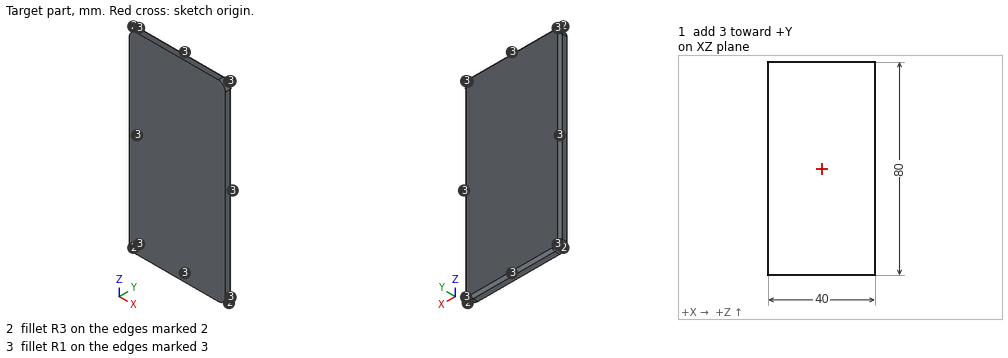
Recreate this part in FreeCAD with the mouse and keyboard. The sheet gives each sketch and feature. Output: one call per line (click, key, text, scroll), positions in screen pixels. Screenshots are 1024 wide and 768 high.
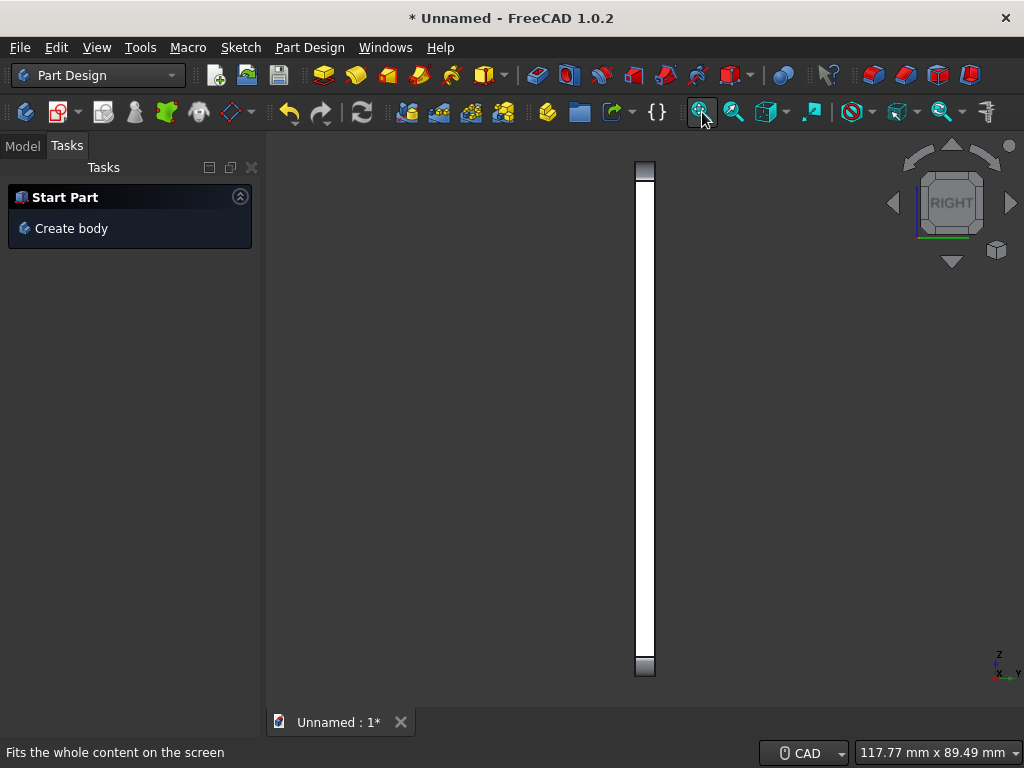
key(5)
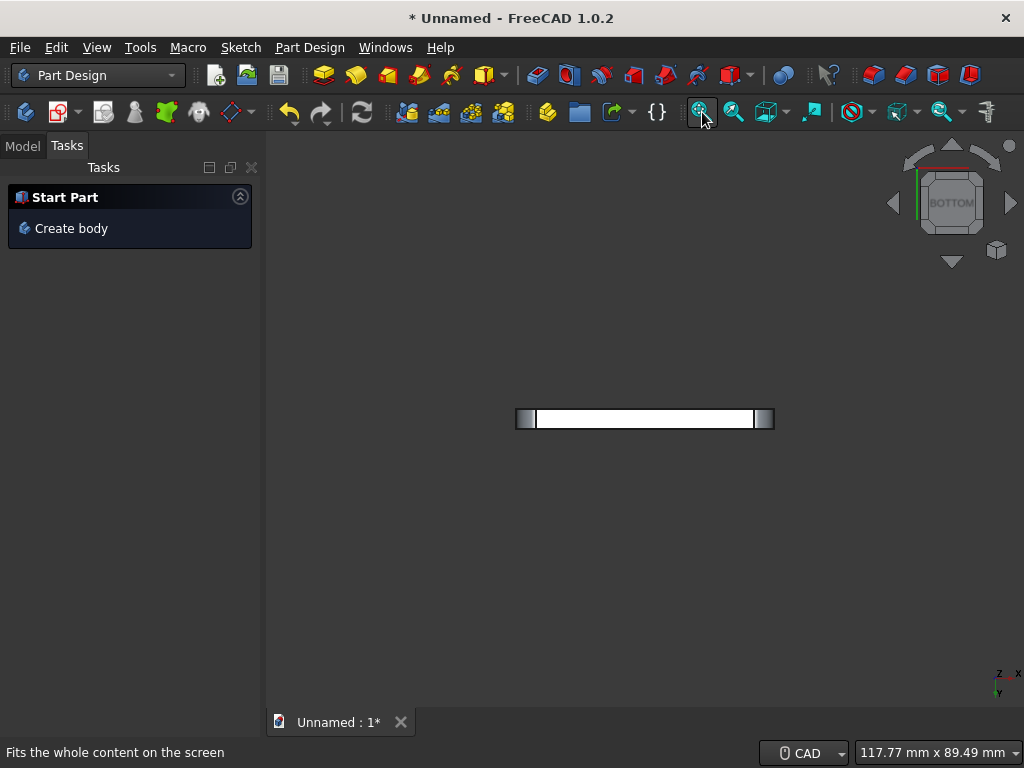
click(702, 112)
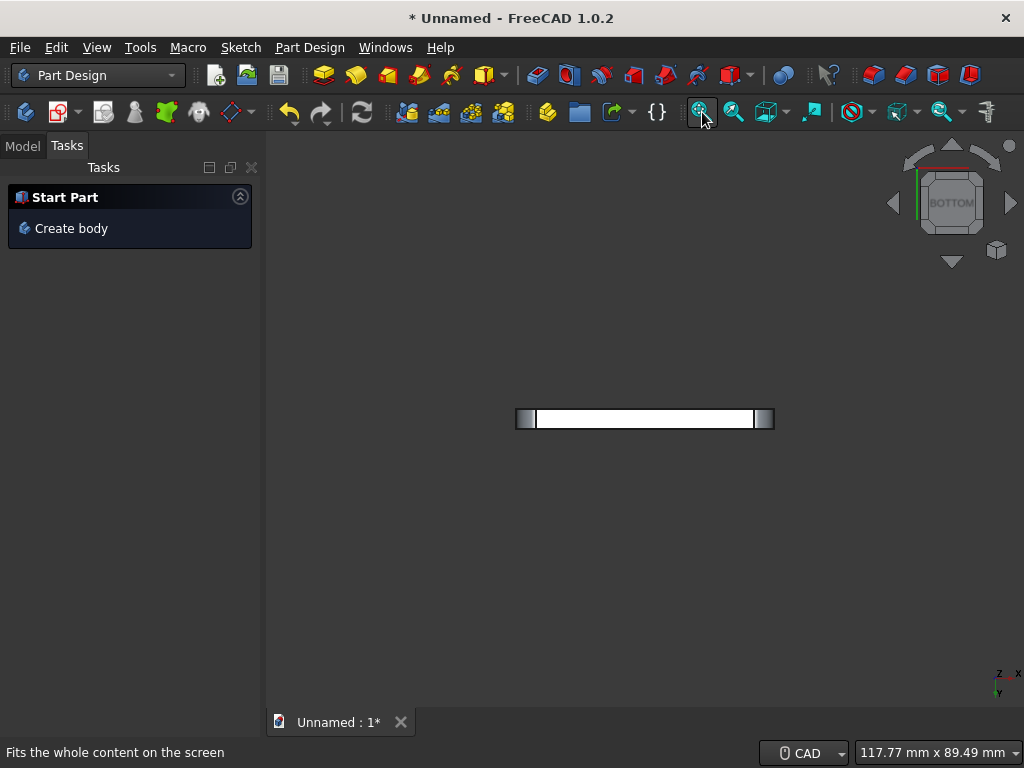
key(4)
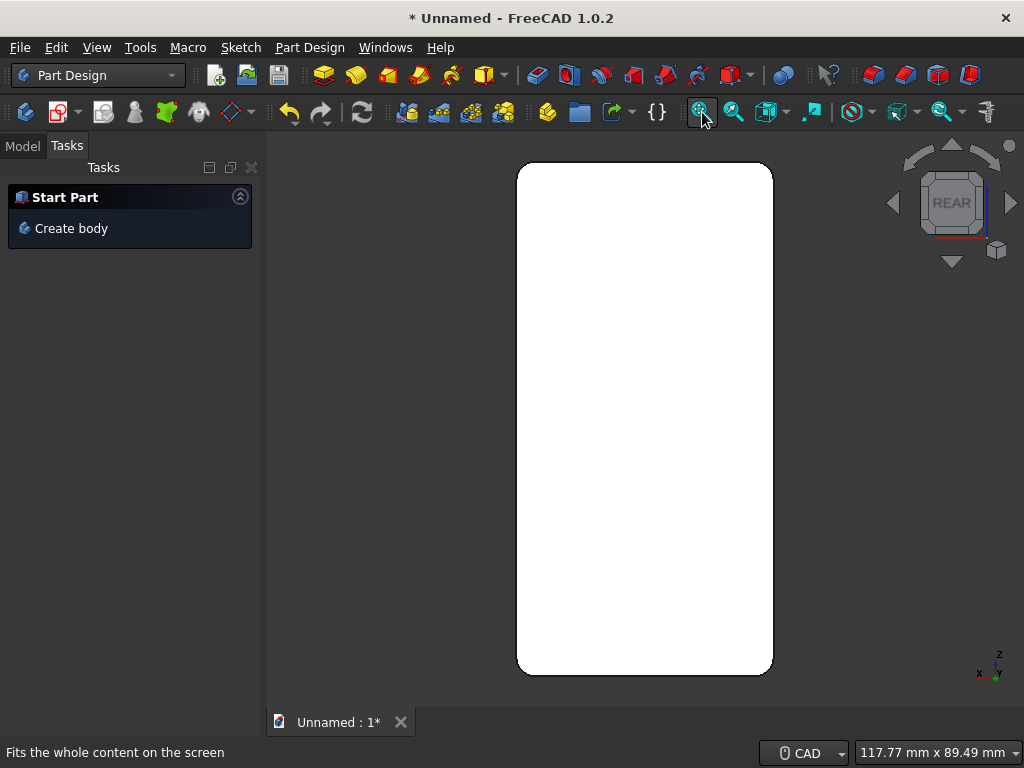
click(645, 344)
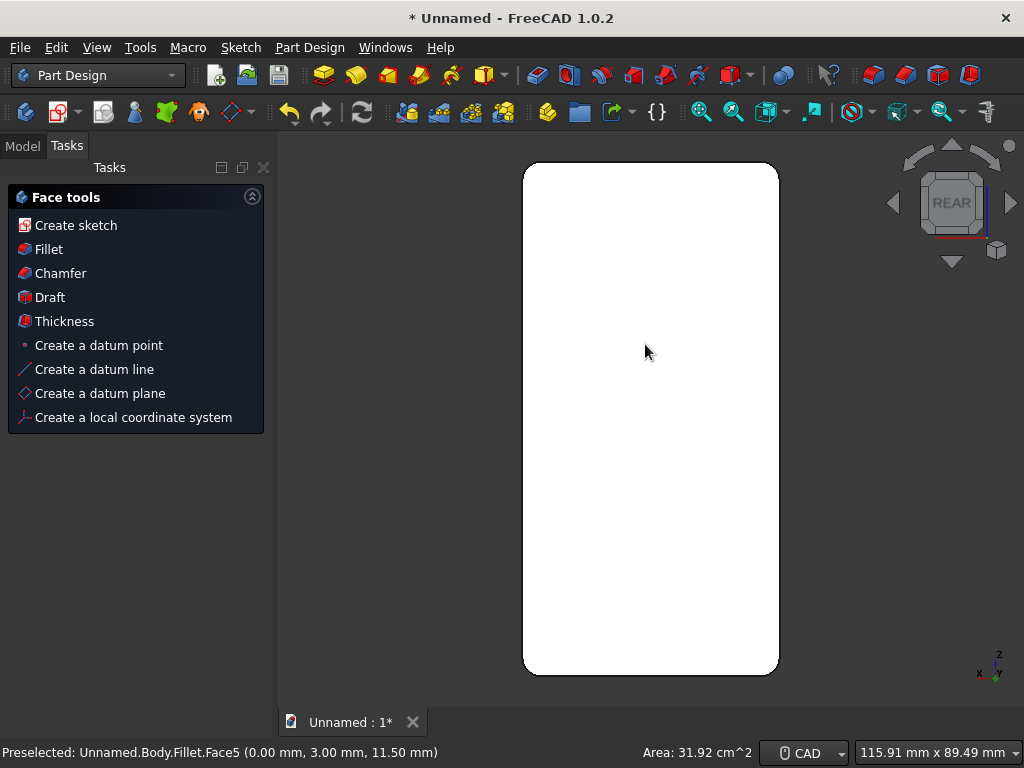
click(874, 76)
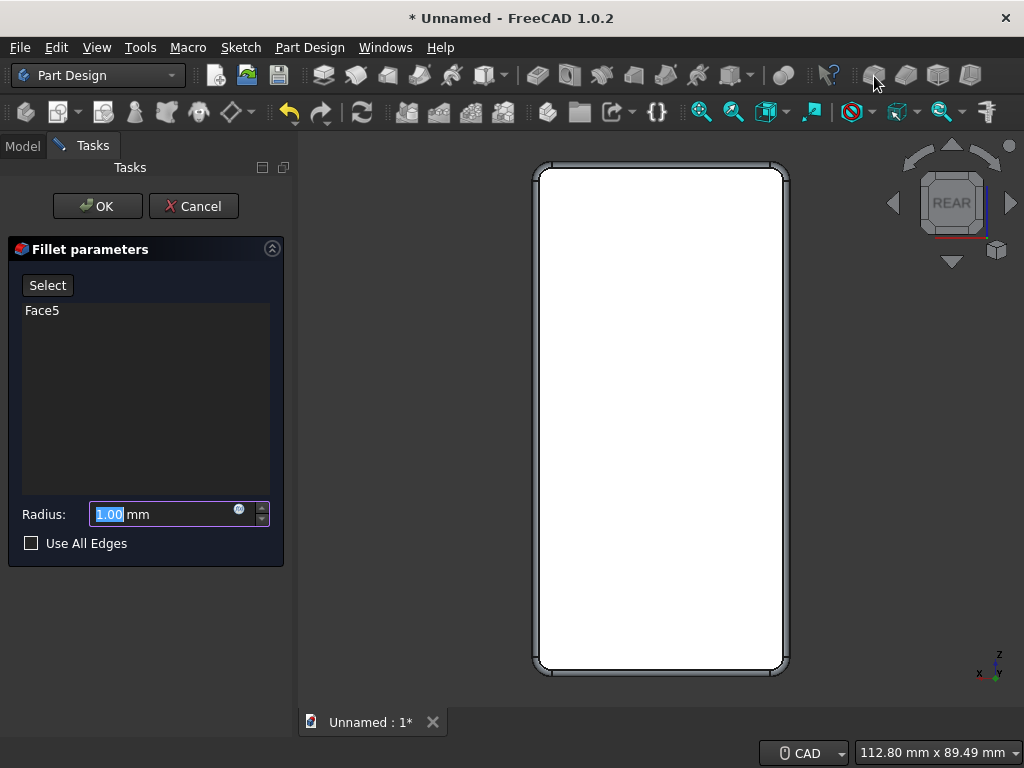
text(1)
key(Tab)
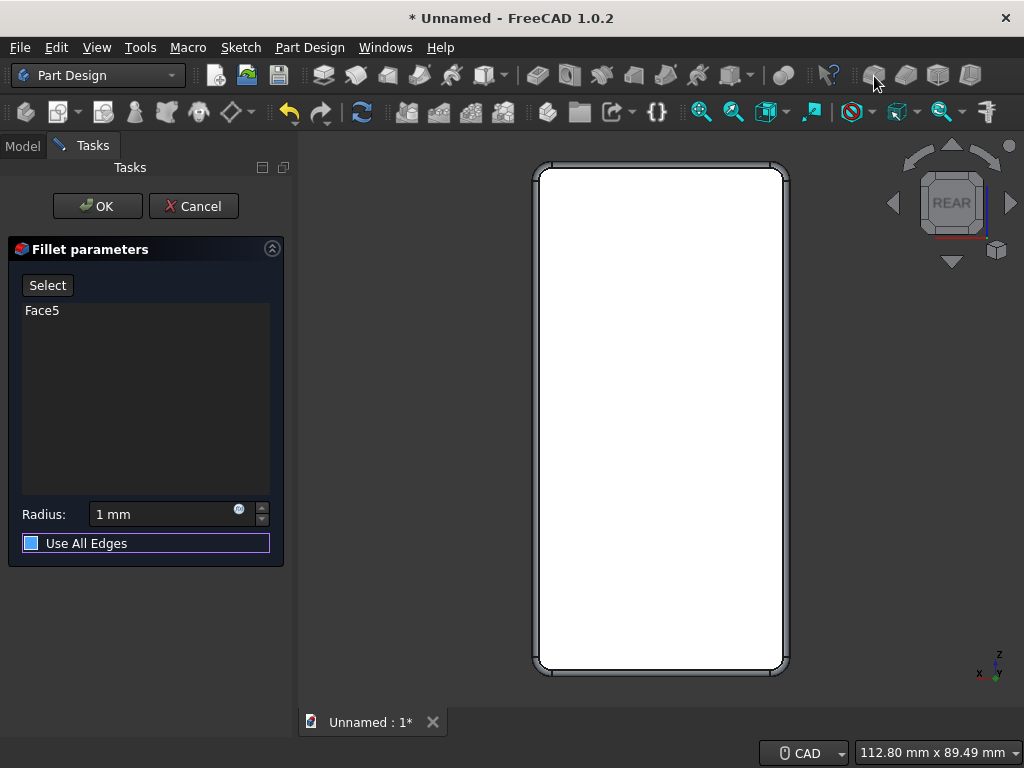
click(98, 206)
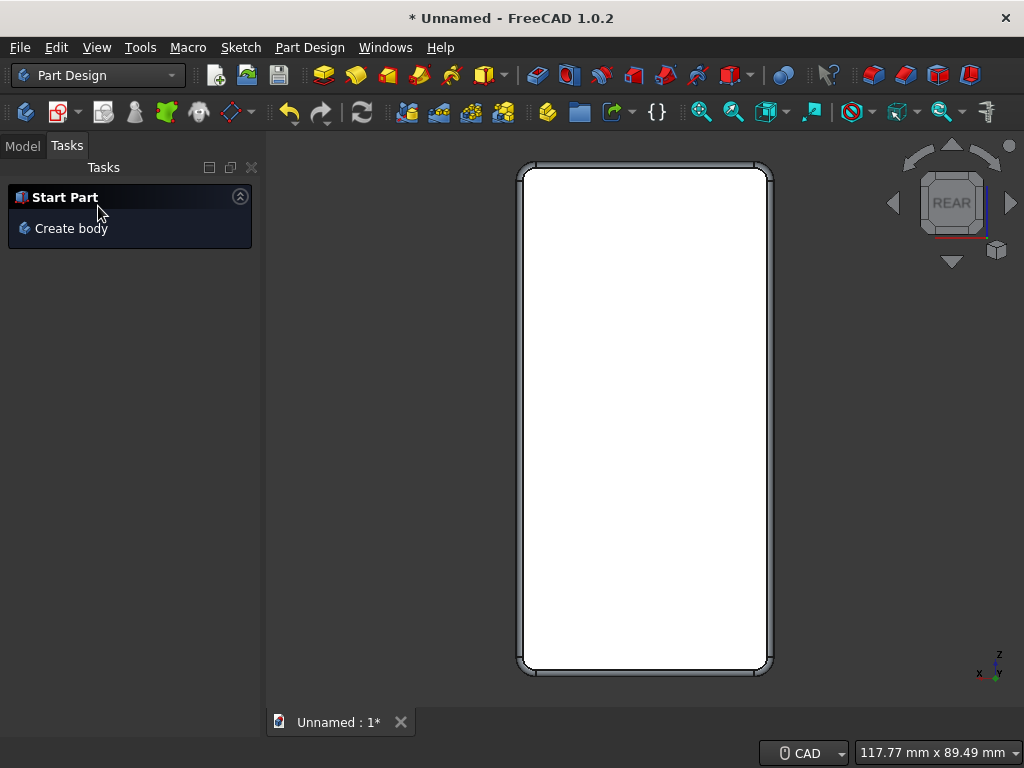
key(0)